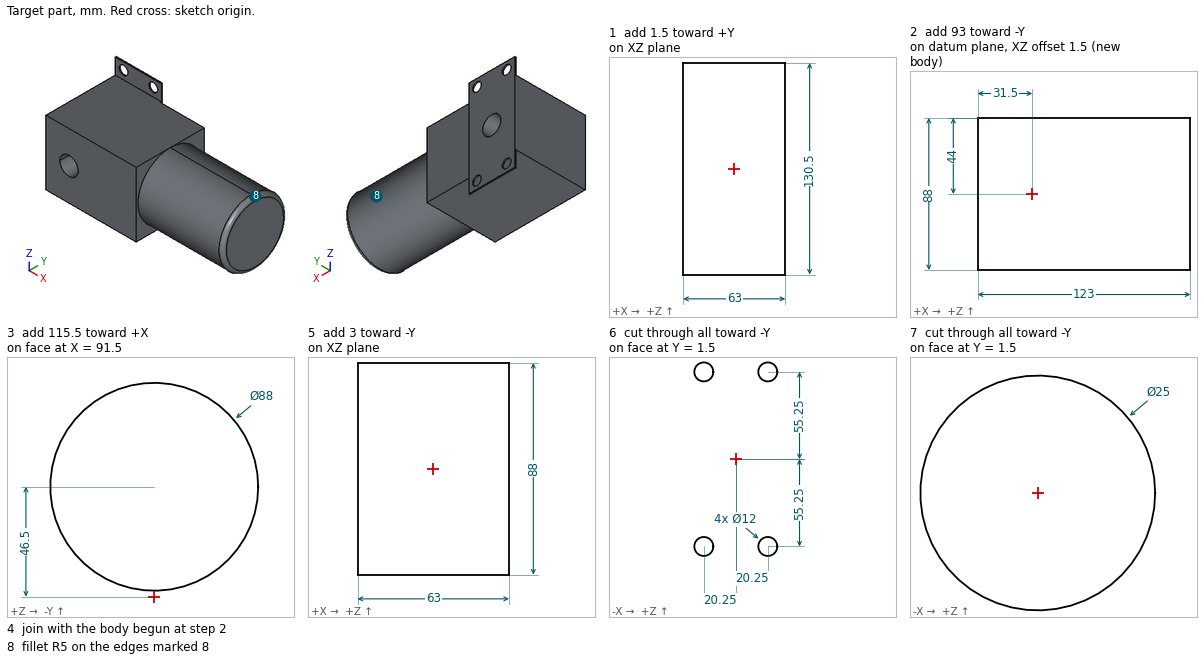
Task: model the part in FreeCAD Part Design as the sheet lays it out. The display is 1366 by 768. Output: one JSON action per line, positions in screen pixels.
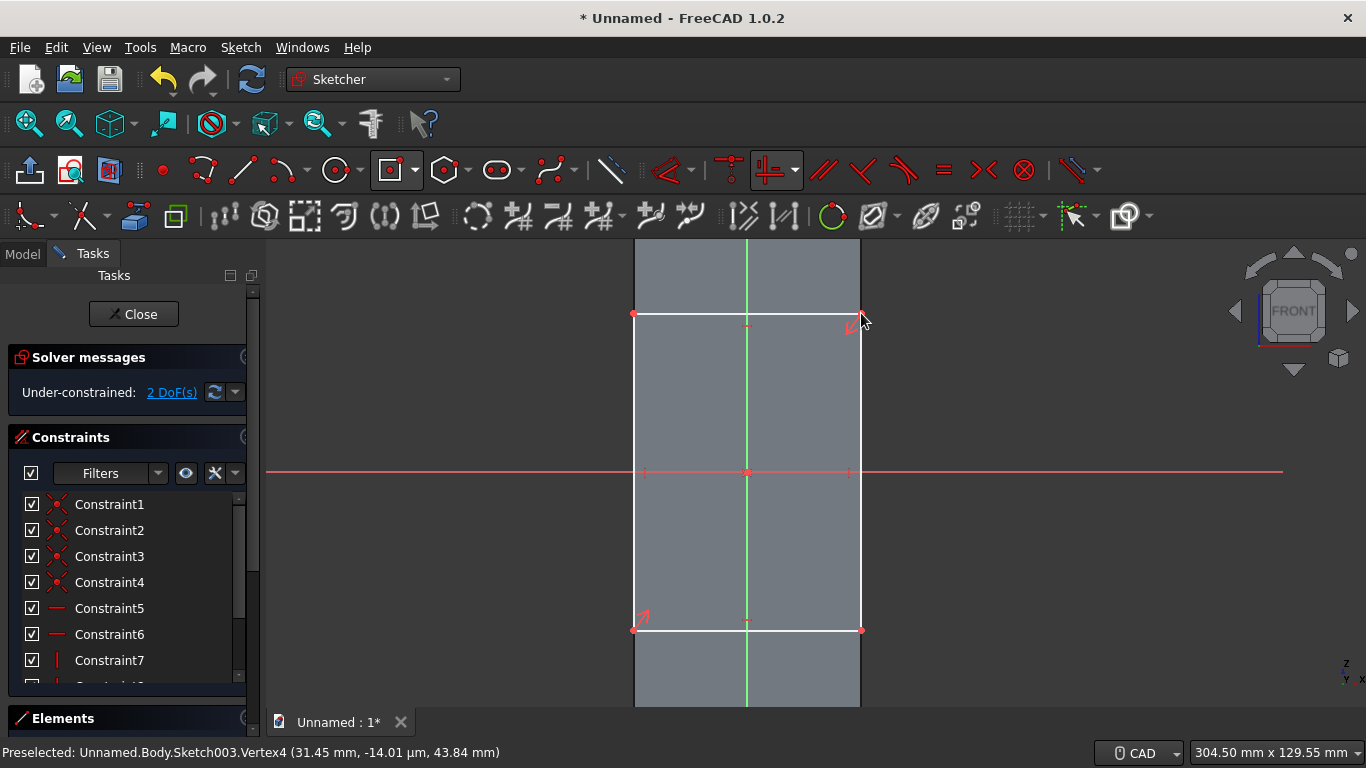
{"action": "left_click", "coordinate": [666, 170]}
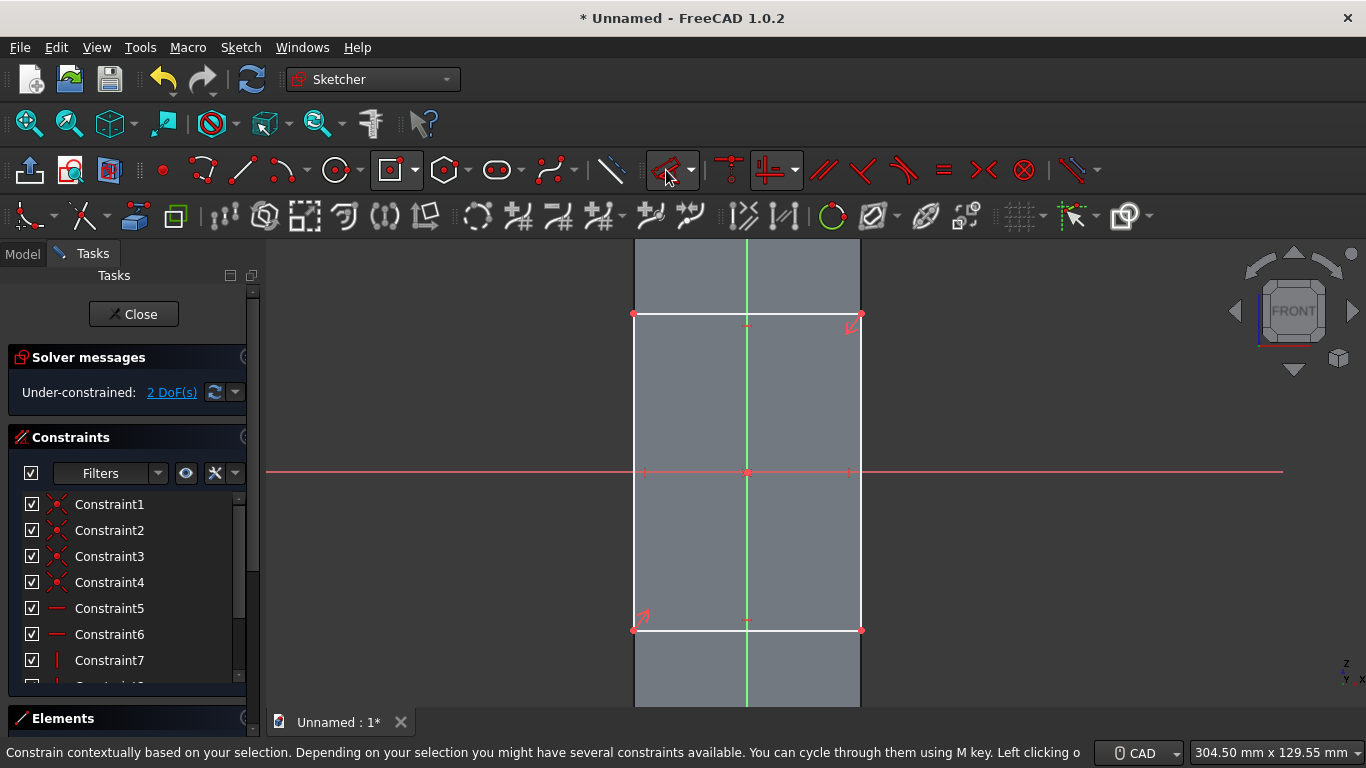
{"action": "left_click", "coordinate": [702, 631]}
{"action": "left_click", "coordinate": [695, 665]}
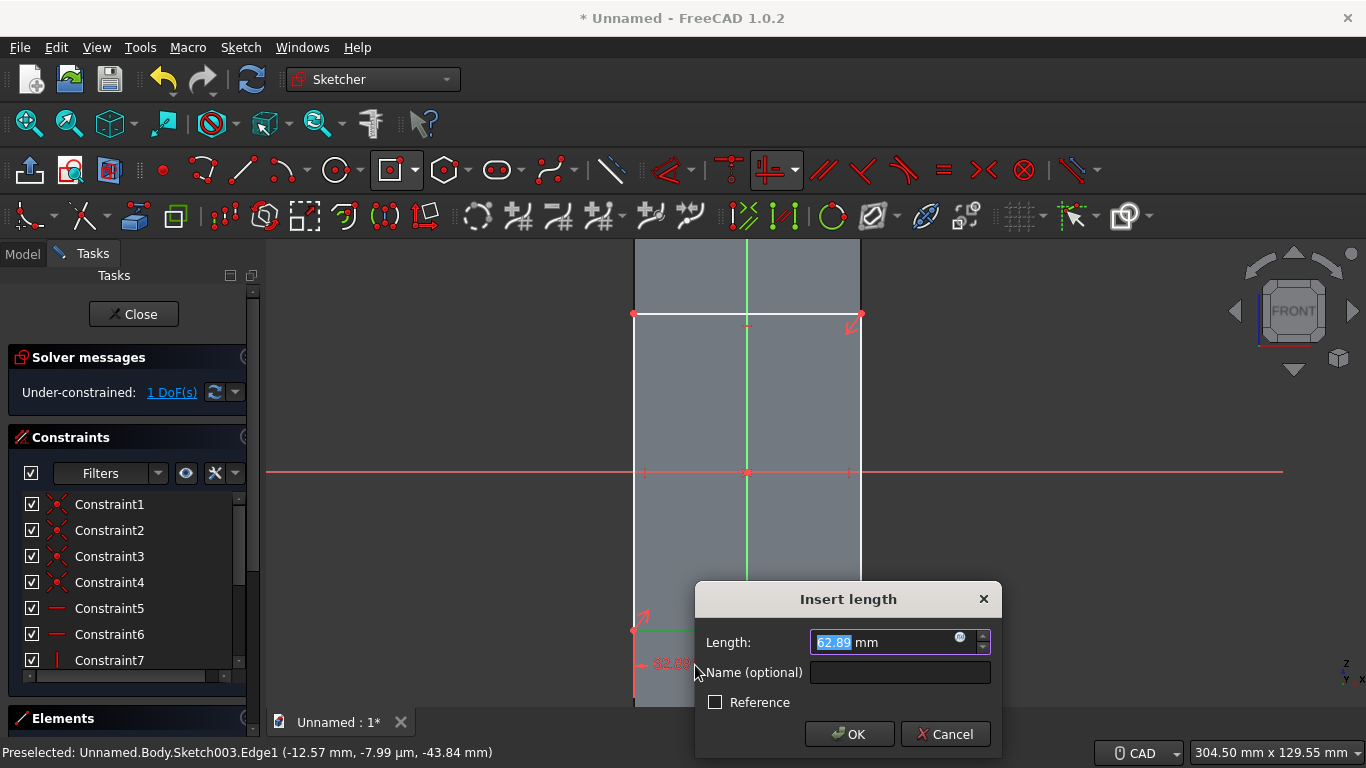
{"action": "type", "text": "63"}
{"action": "key", "text": "Return"}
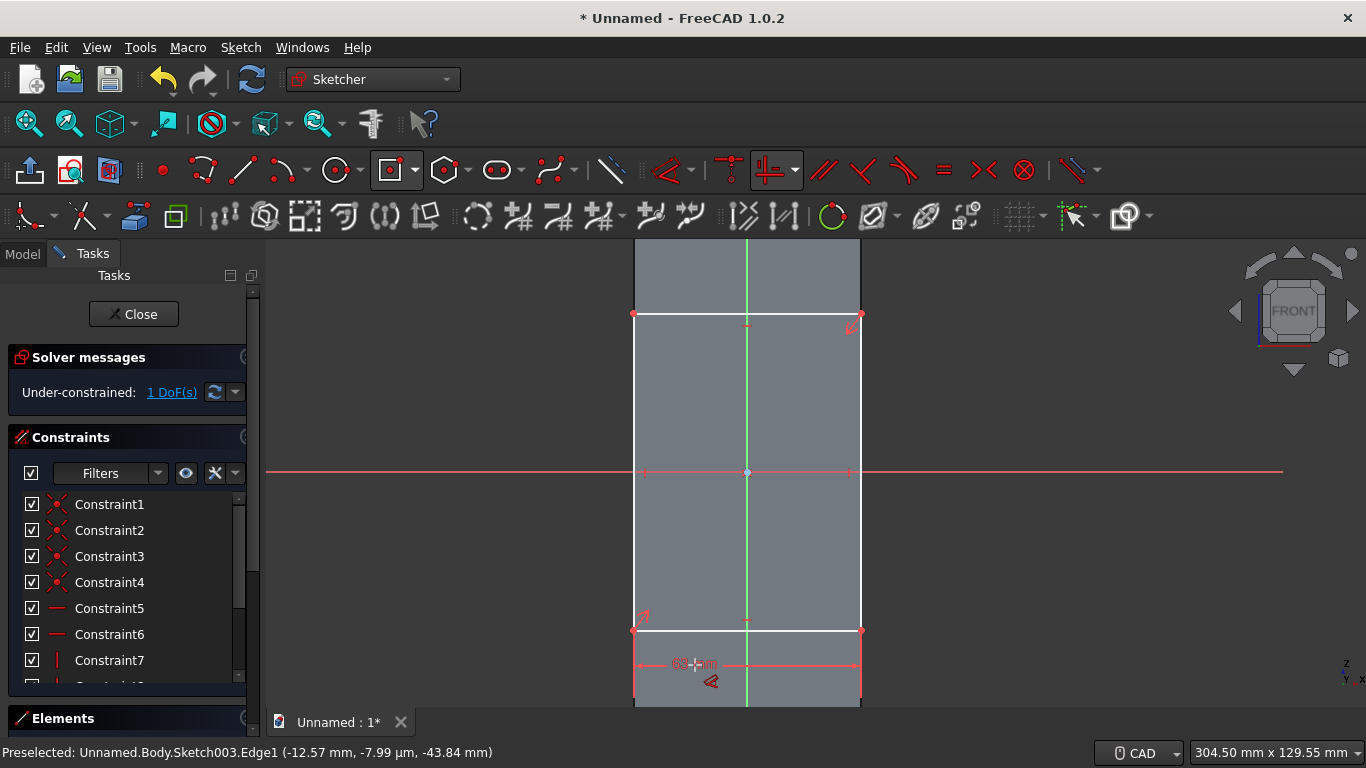
{"action": "left_click", "coordinate": [861, 536]}
{"action": "left_click", "coordinate": [895, 400]}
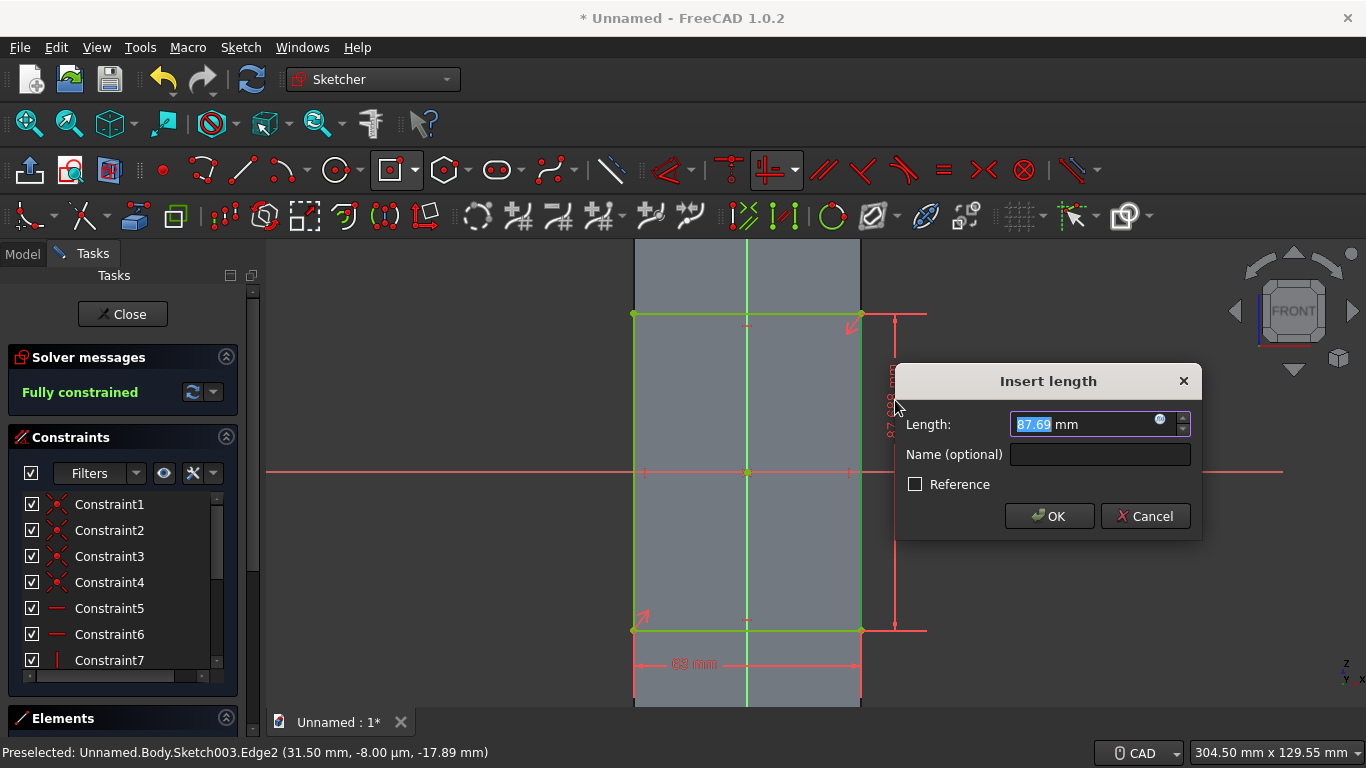
{"action": "type", "text": "88"}
{"action": "key", "text": "Return"}
{"action": "key", "text": "Escape"}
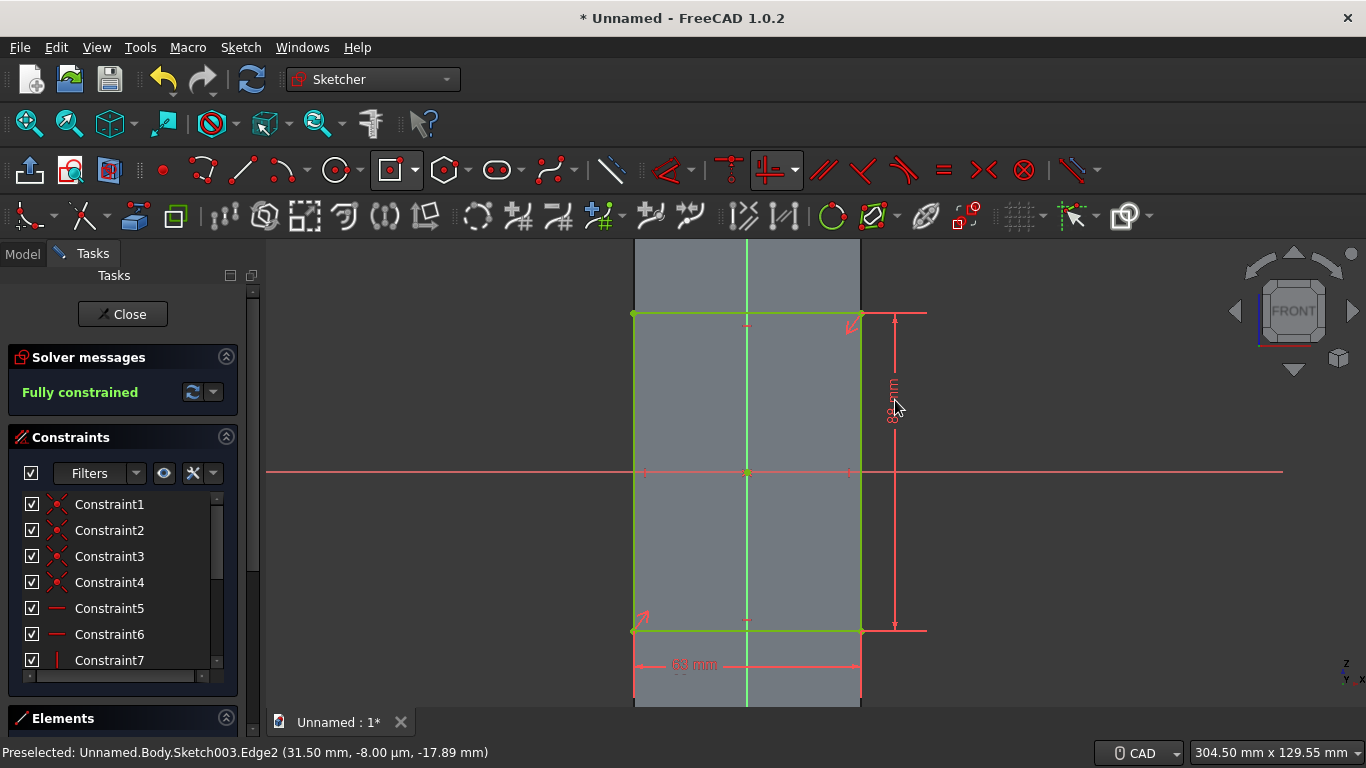
{"action": "left_click", "coordinate": [123, 314]}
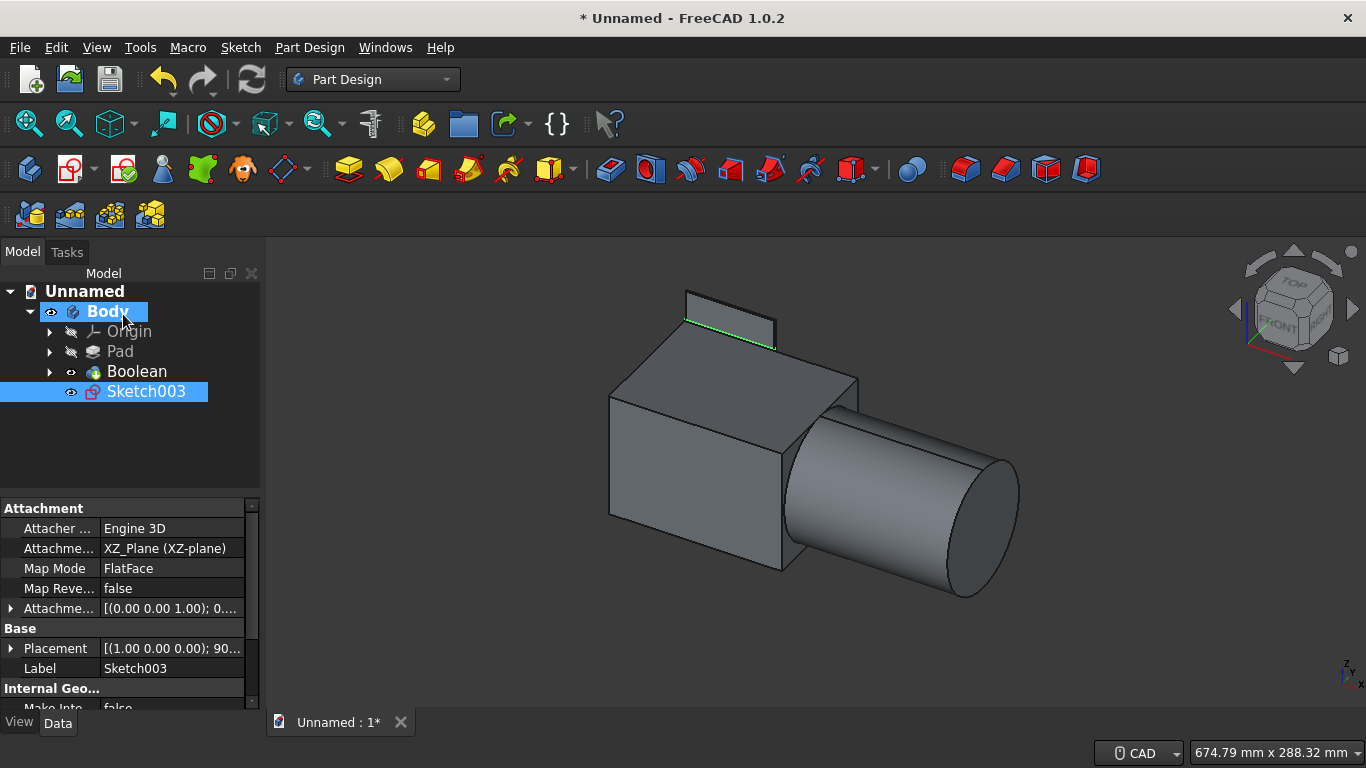
{"action": "left_click", "coordinate": [350, 170]}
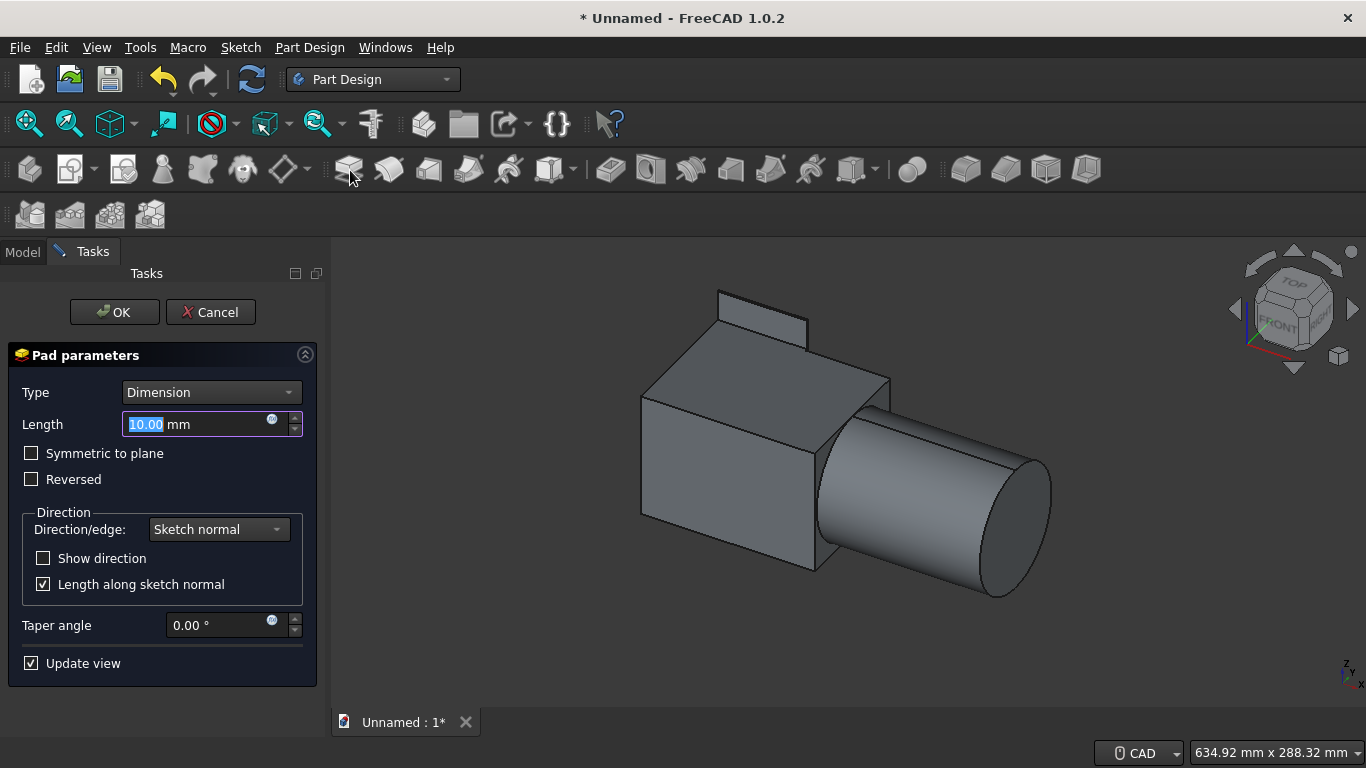
{"action": "type", "text": "3"}
{"action": "key", "text": "Tab"}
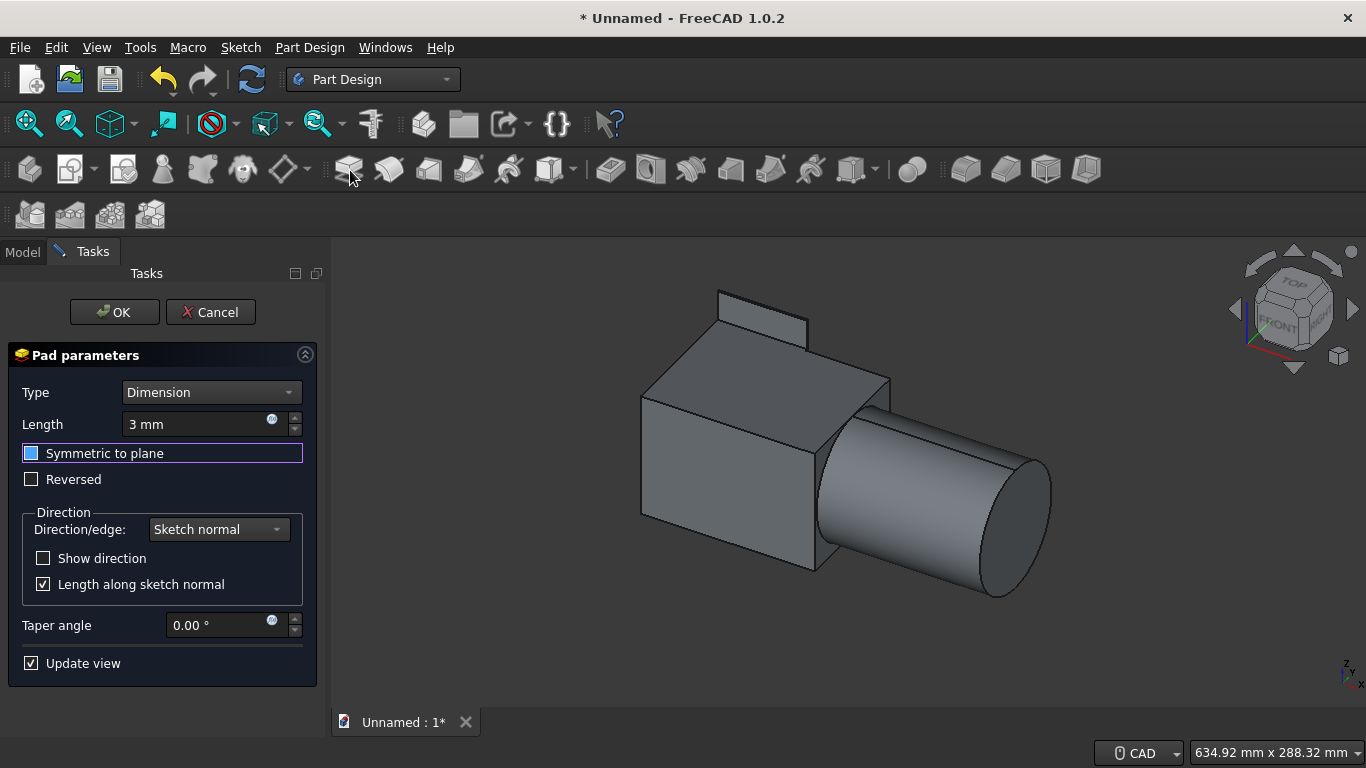
{"action": "left_click", "coordinate": [115, 312]}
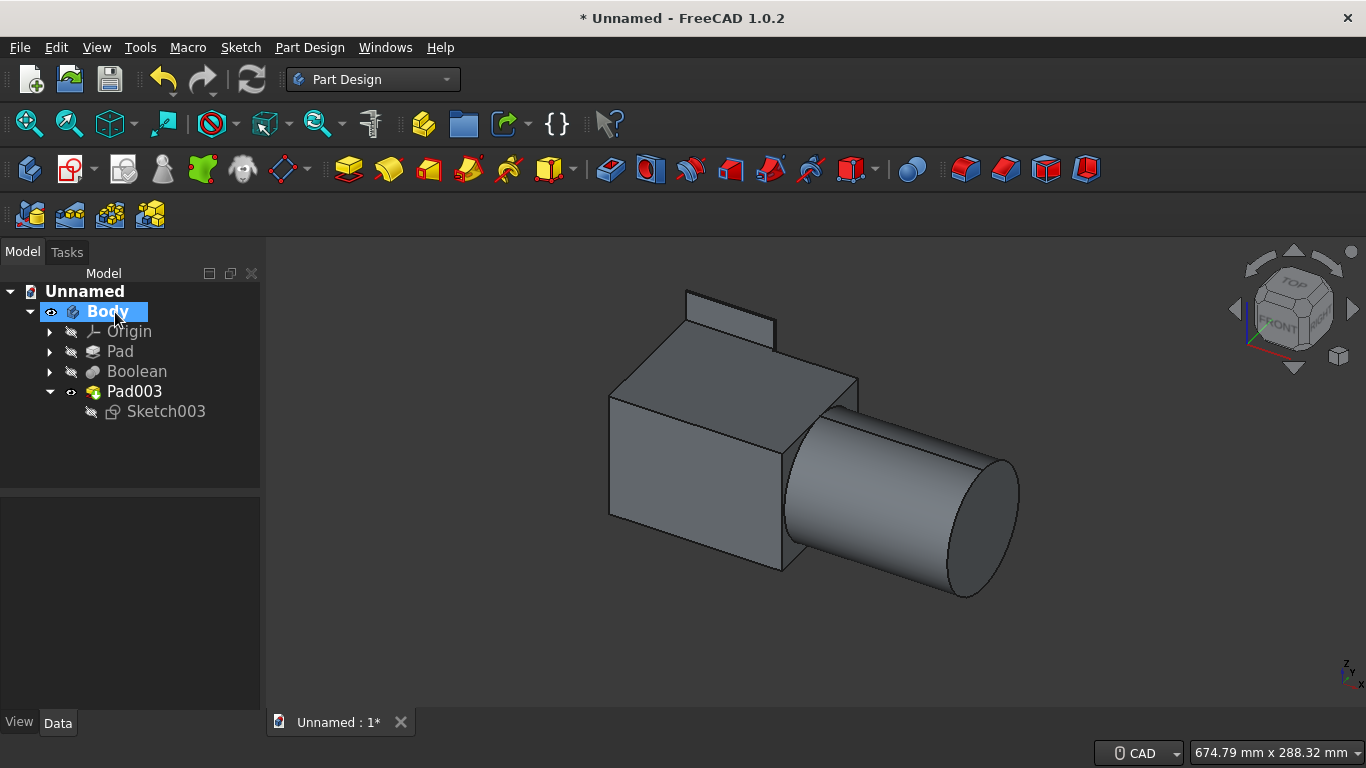
{"action": "key", "text": "4"}